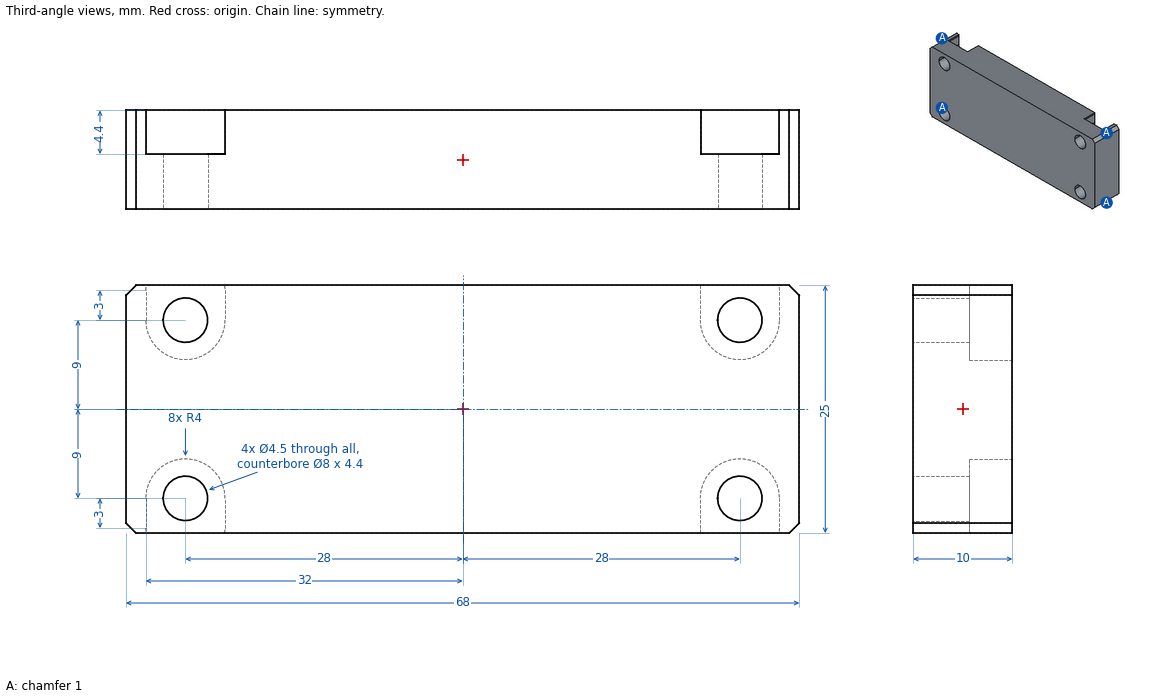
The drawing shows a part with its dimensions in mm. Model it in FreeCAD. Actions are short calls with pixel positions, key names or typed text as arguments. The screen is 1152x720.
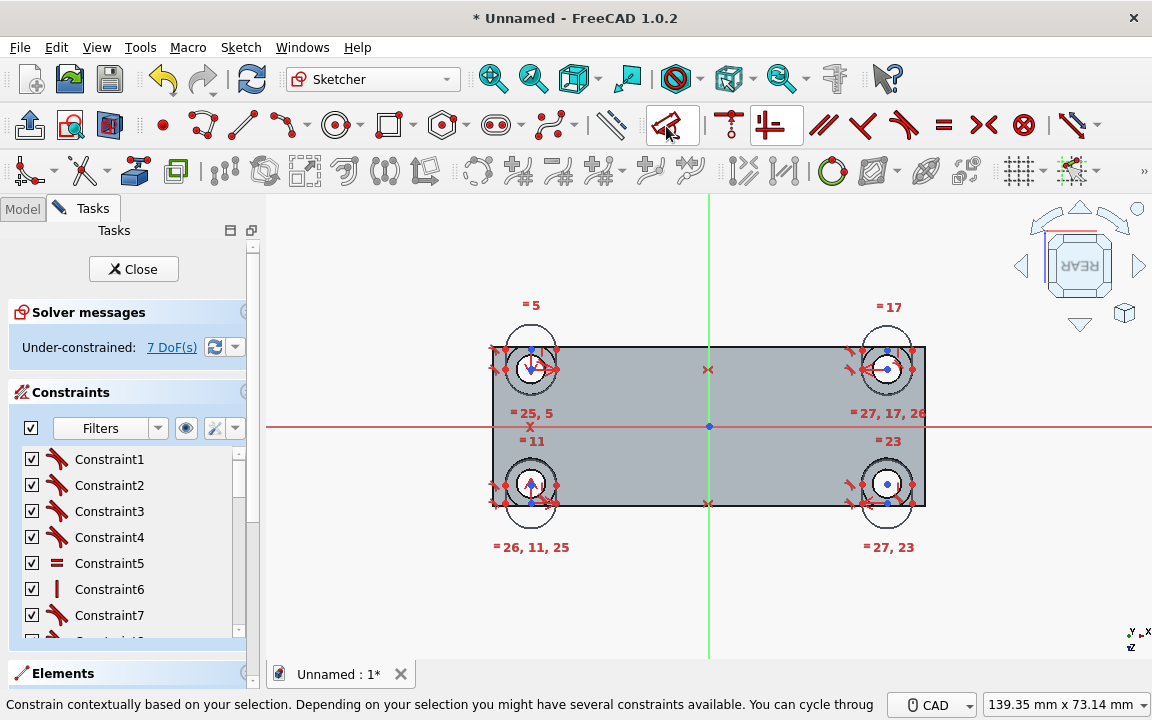
scroll(516, 390, up, 3)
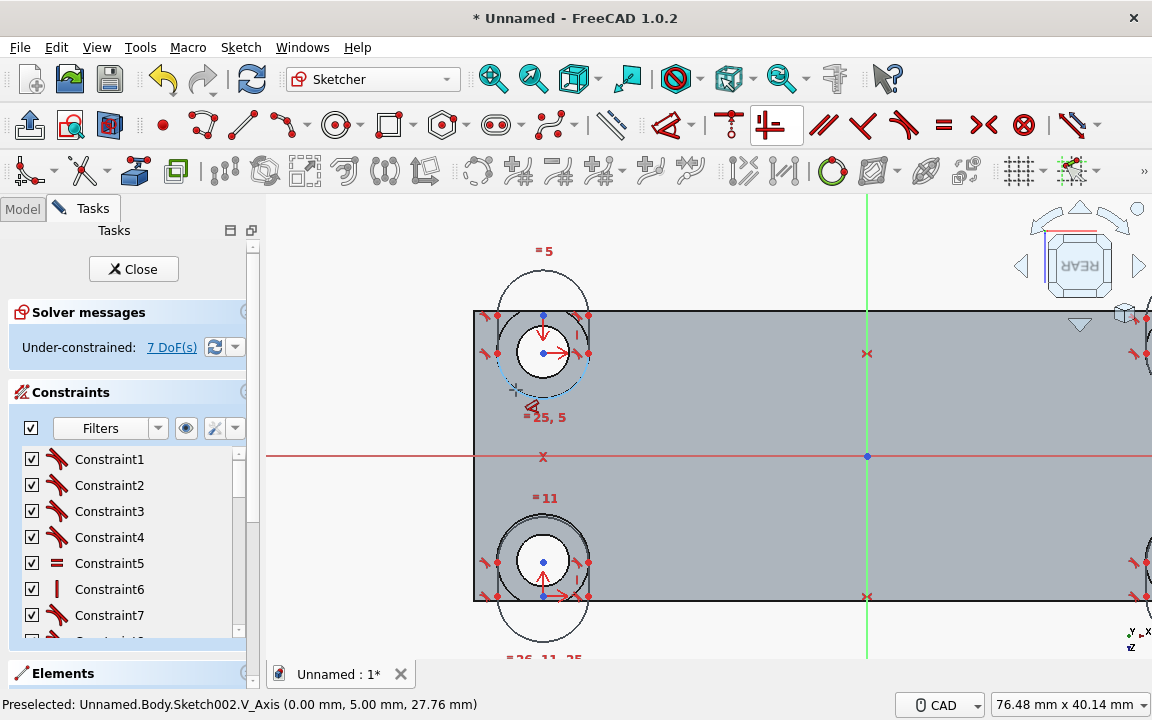
click(516, 390)
click(497, 416)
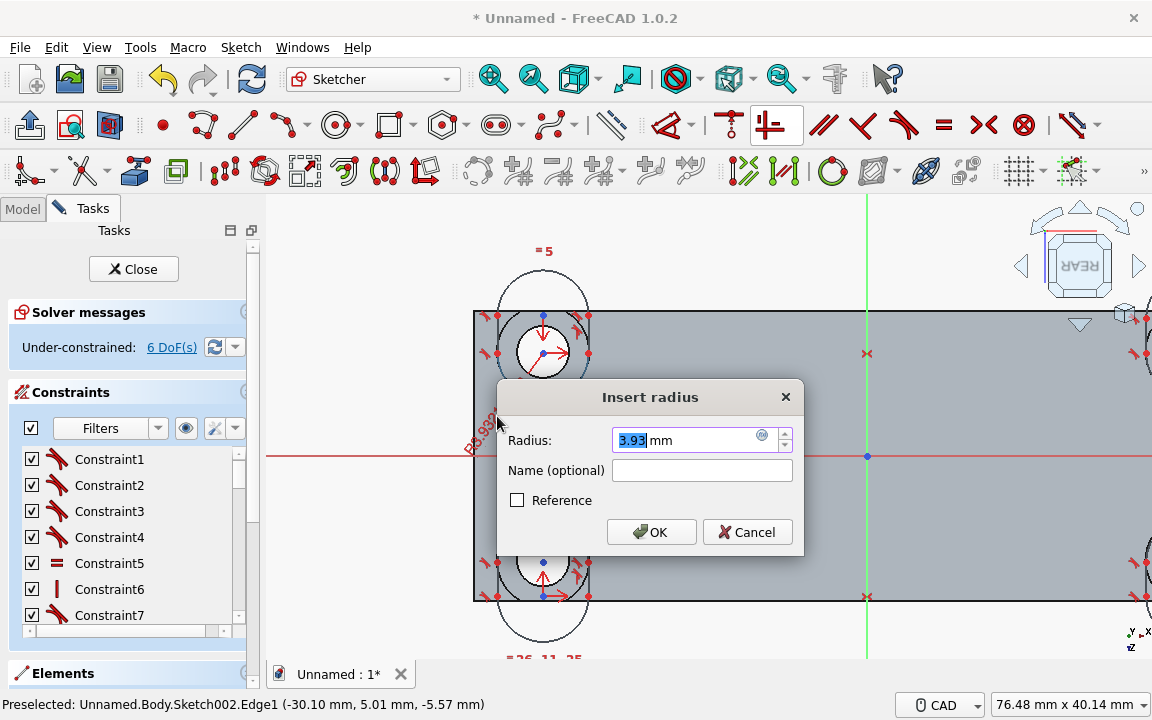
text(4)
key(Return)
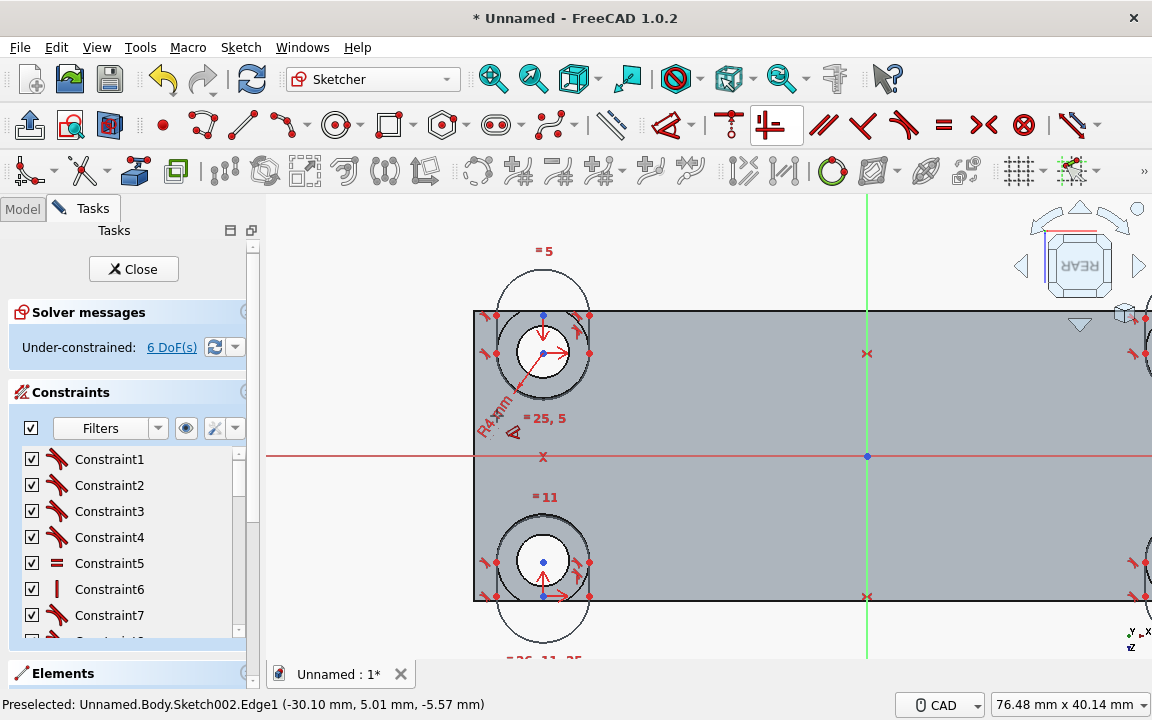
scroll(497, 342, up, 2)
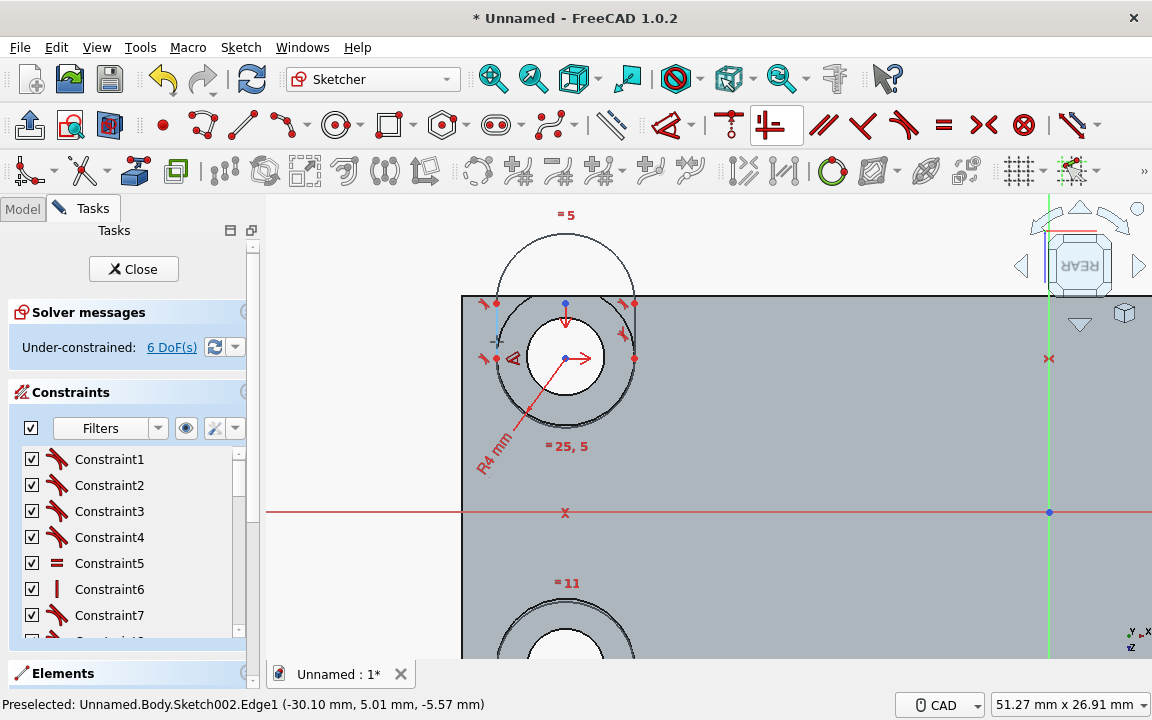
click(497, 342)
click(463, 331)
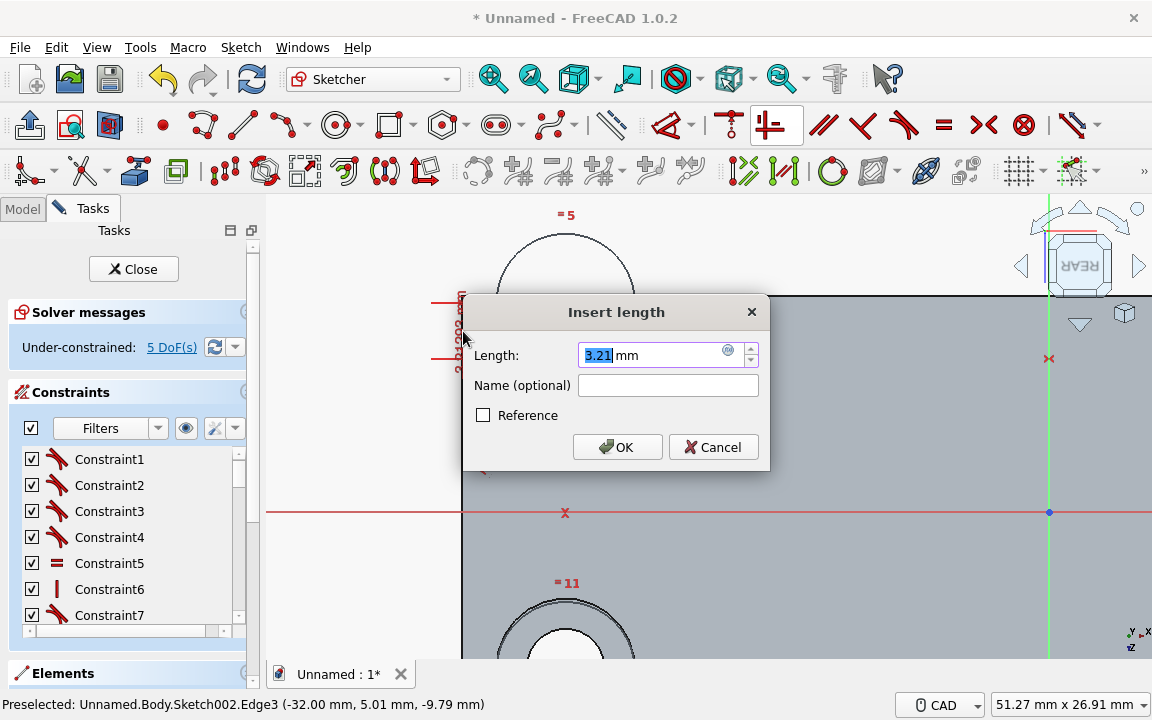
text(3)
key(Return)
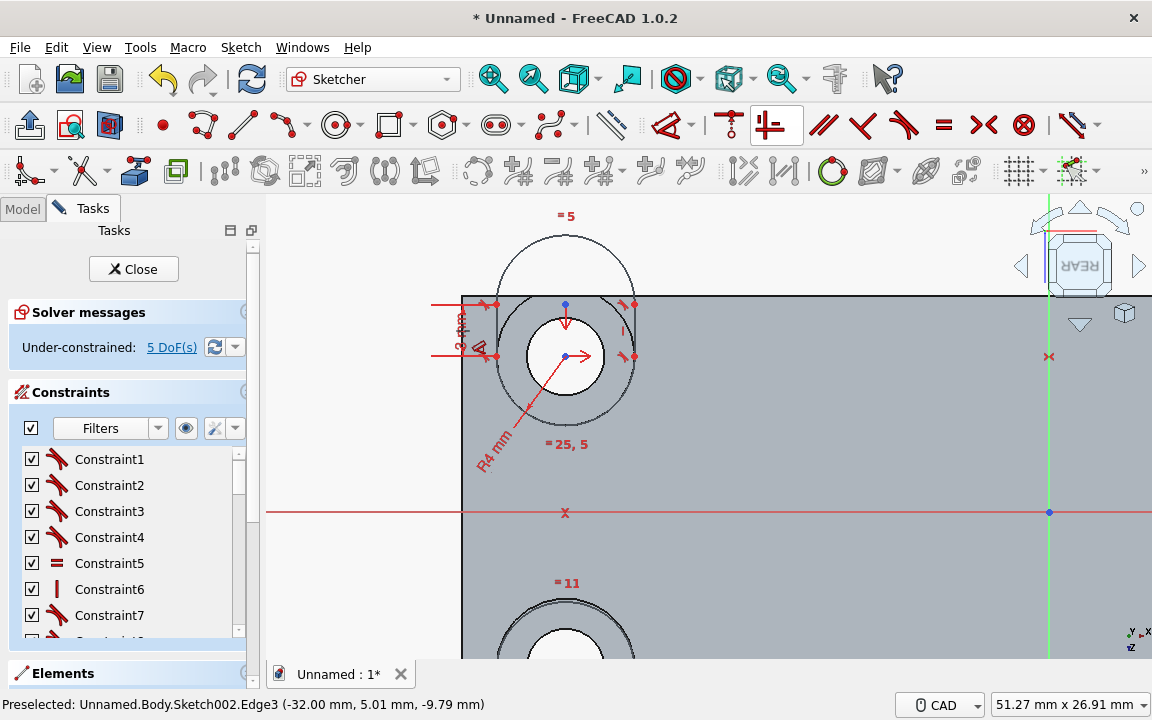
scroll(307, 357, down, 4)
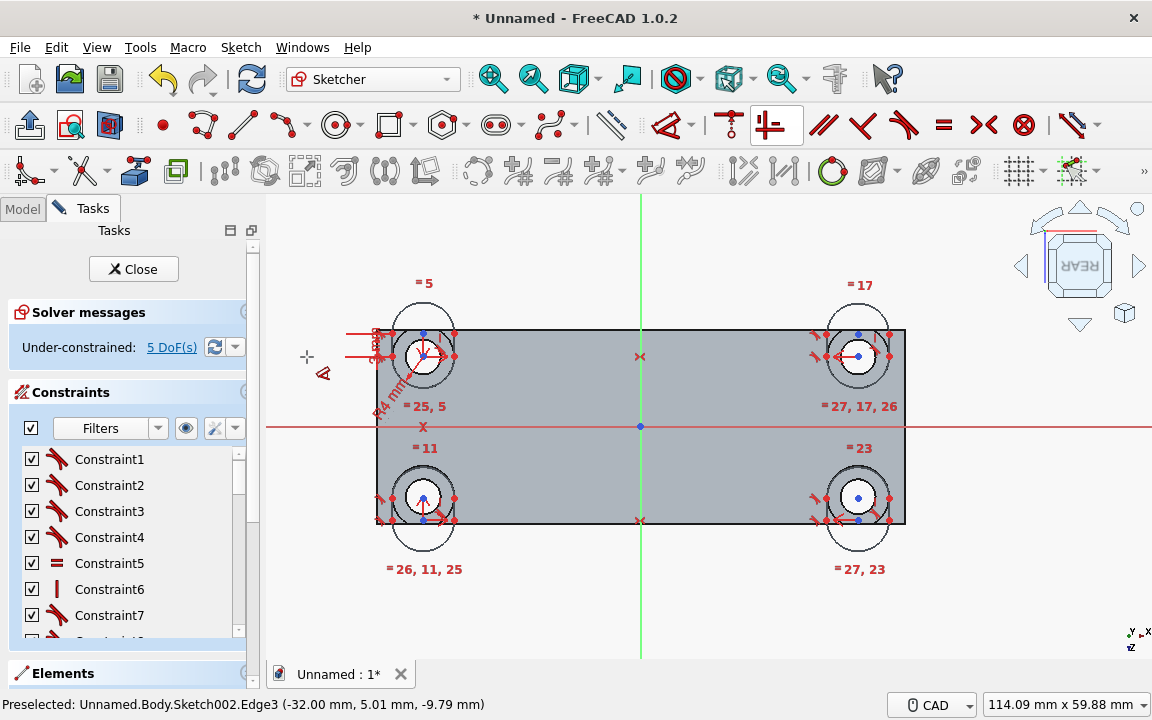
scroll(392, 514, up, 4)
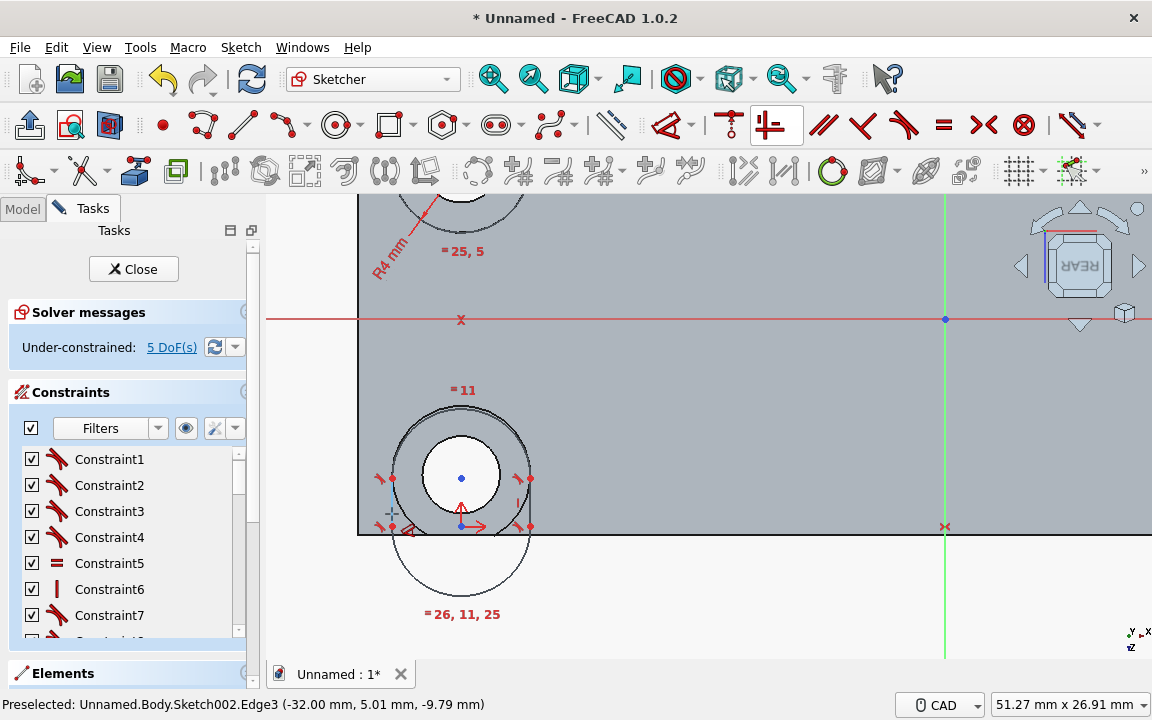
click(392, 512)
click(358, 503)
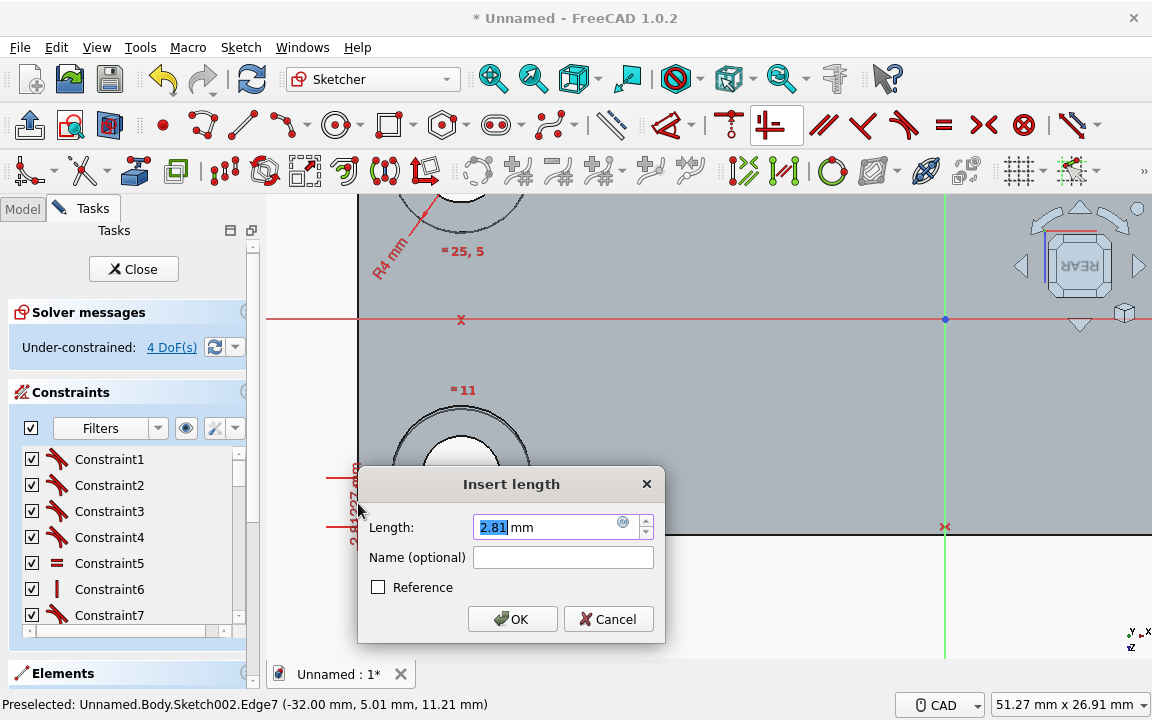
text(3)
key(Return)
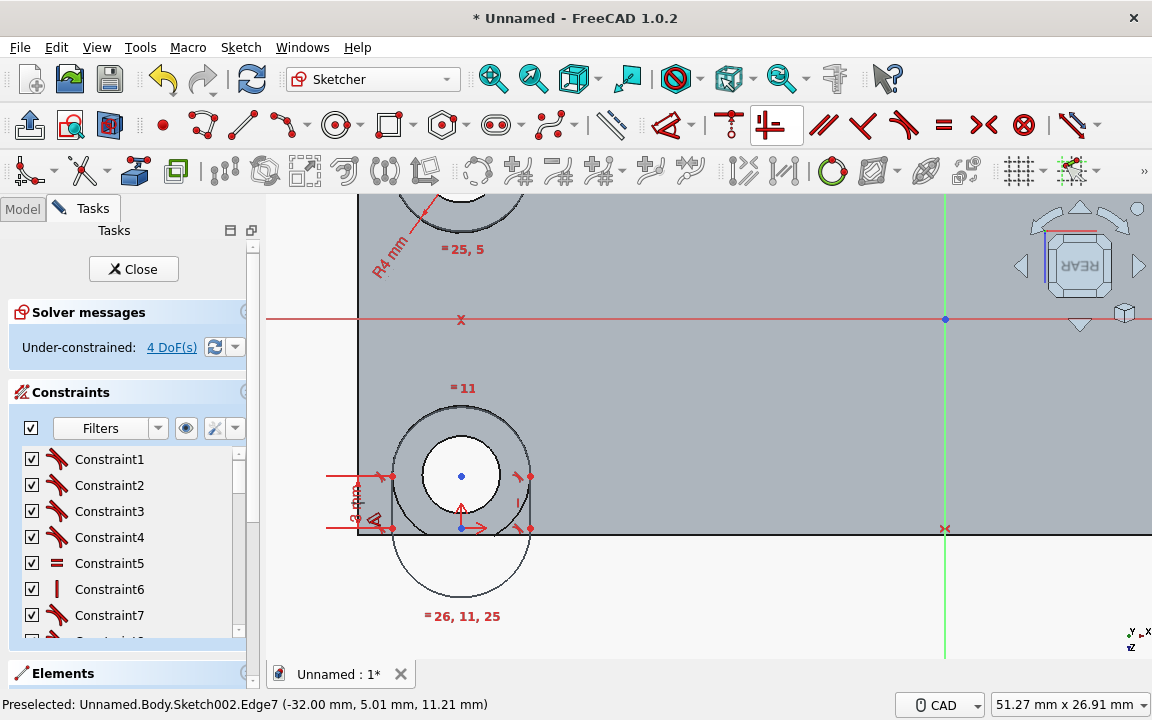
scroll(392, 514, down, 4)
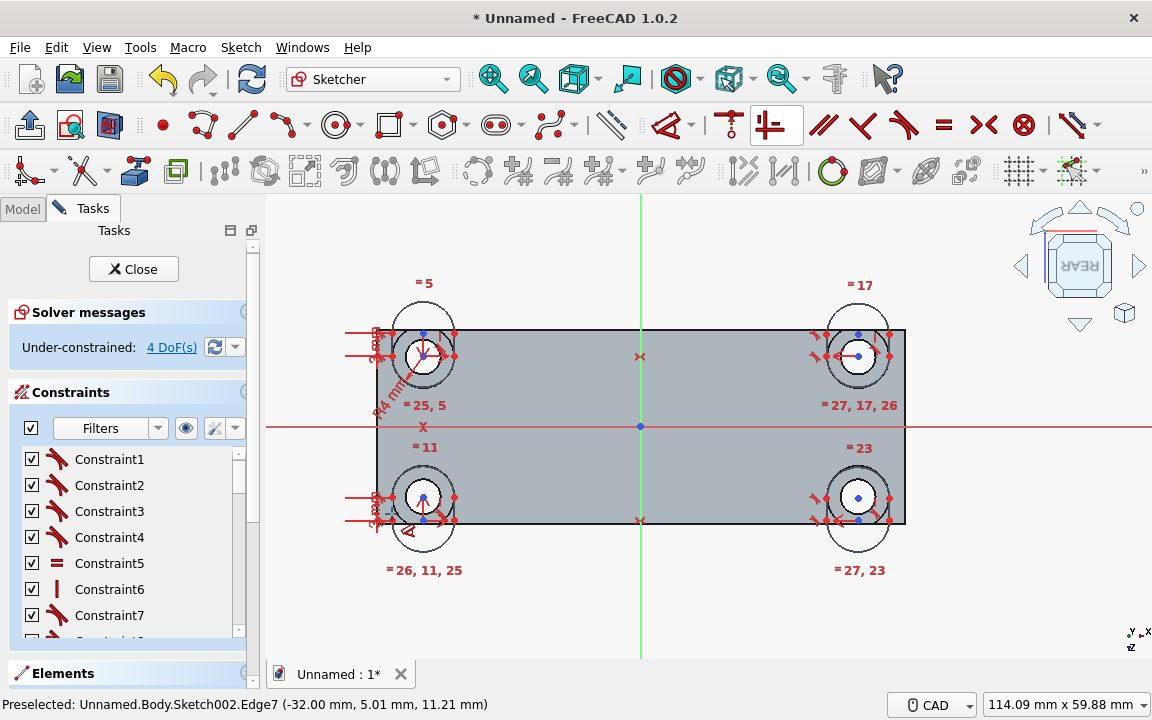
scroll(827, 350, up, 4)